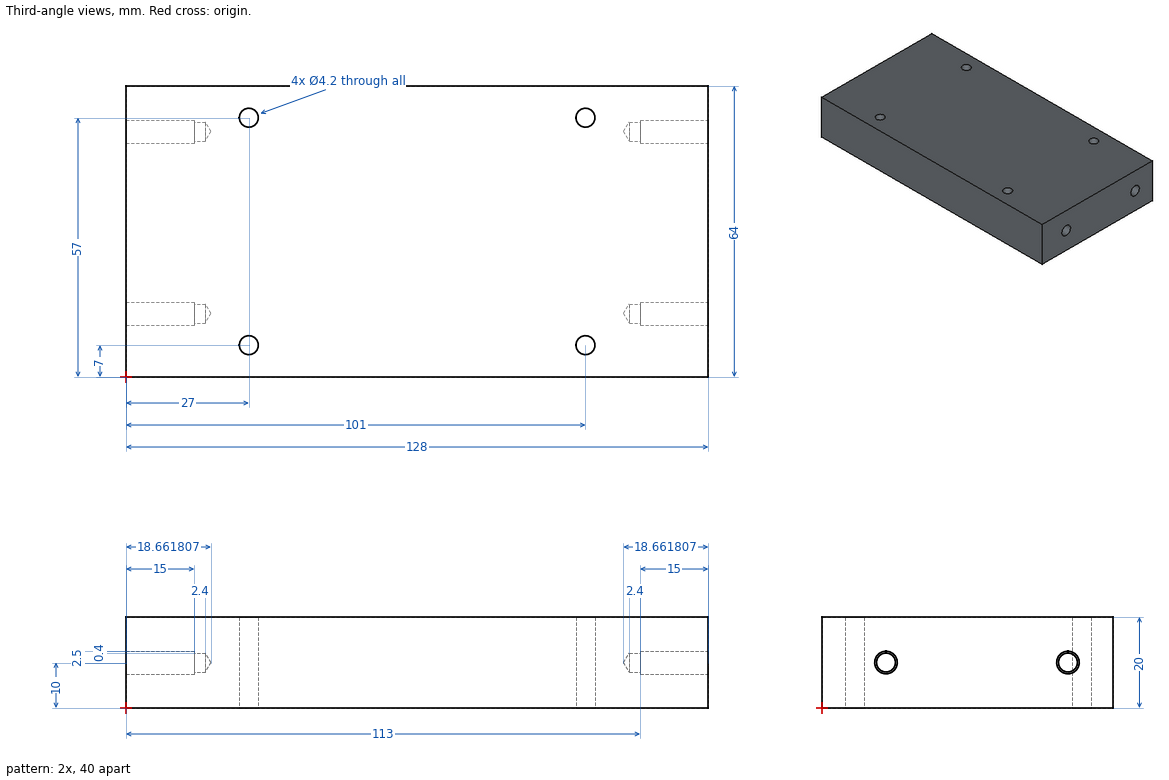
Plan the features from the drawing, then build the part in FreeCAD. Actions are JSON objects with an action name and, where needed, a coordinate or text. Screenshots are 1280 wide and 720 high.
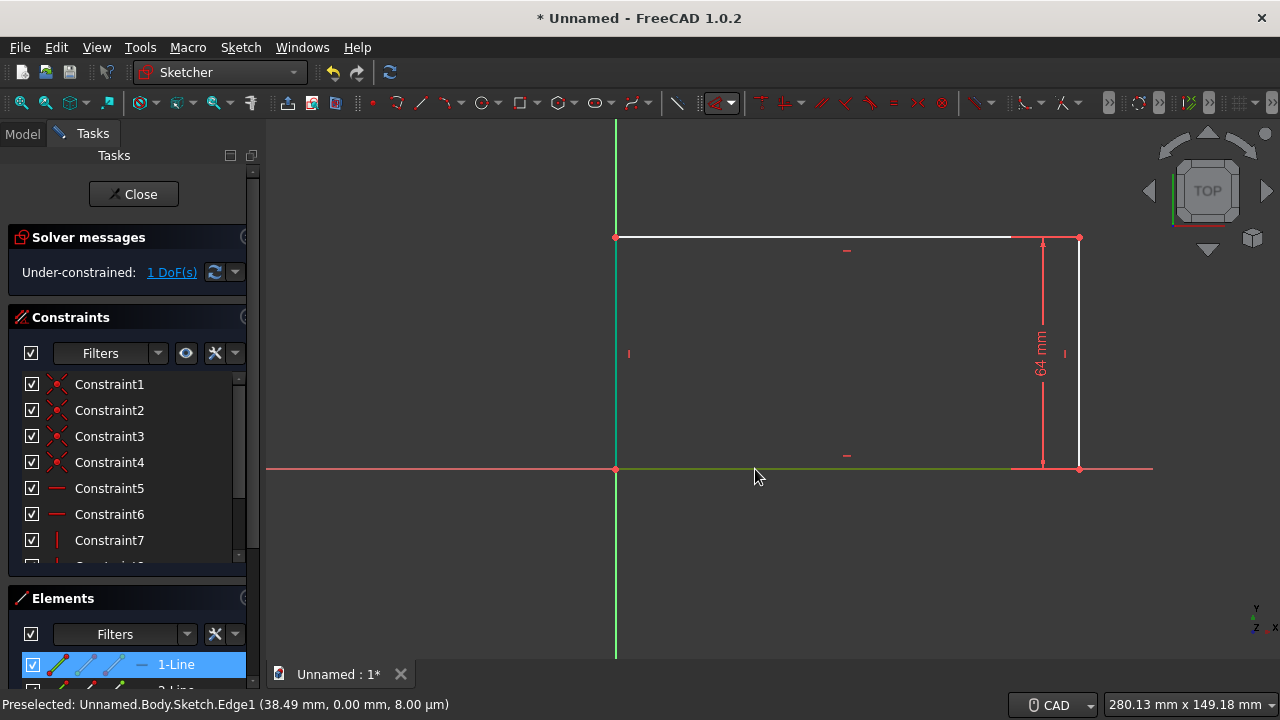
{"action": "left_click", "coordinate": [734, 104]}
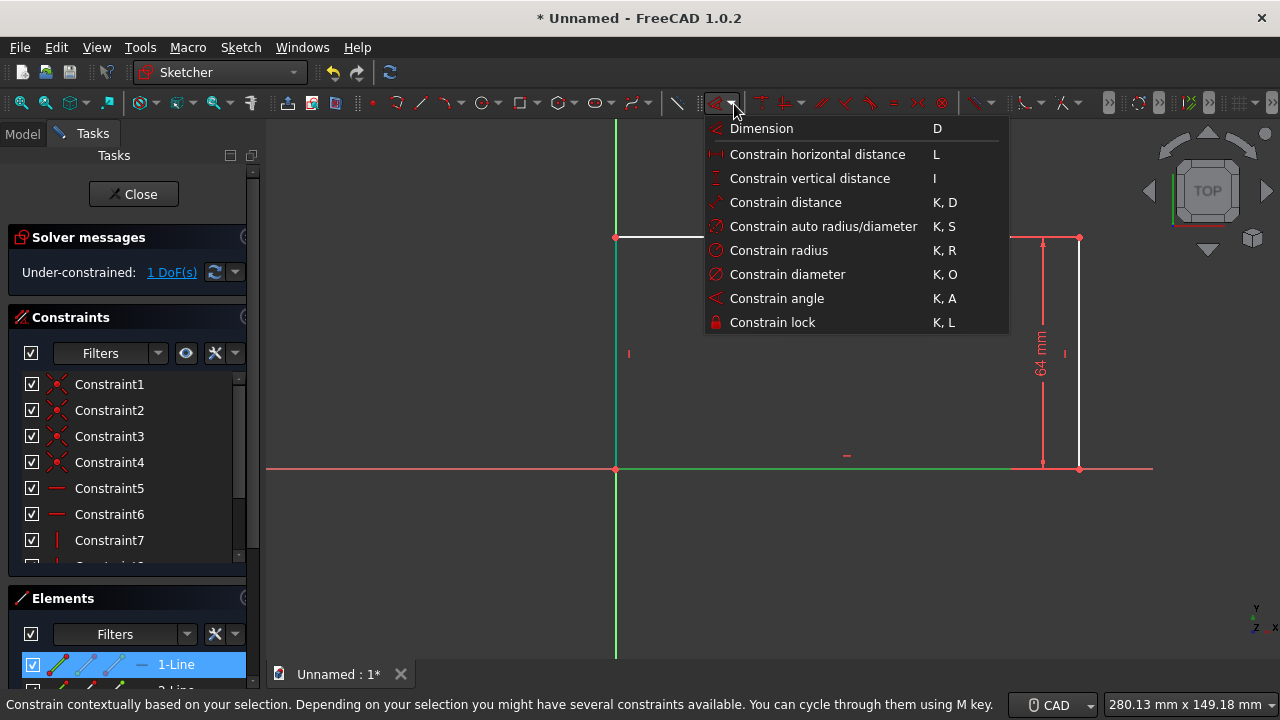
{"action": "left_click", "coordinate": [857, 154]}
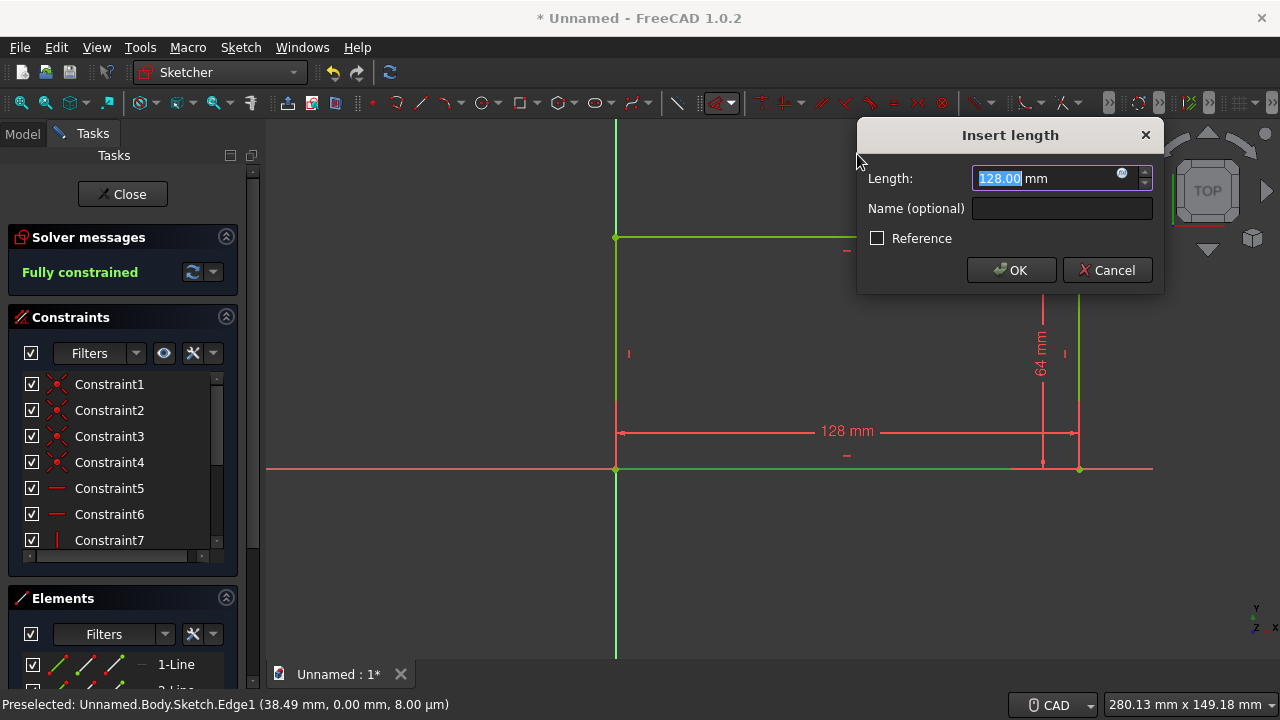
{"action": "type", "text": "128"}
{"action": "key", "text": "Return"}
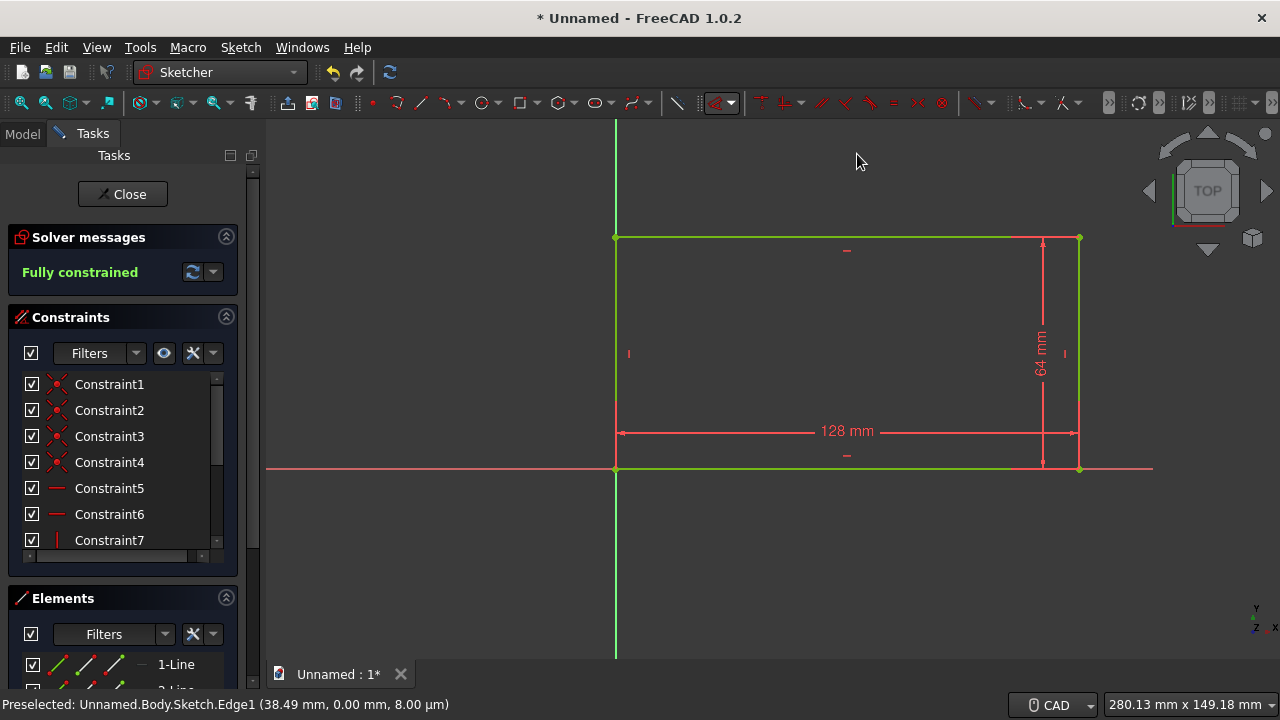
{"action": "left_click", "coordinate": [123, 194]}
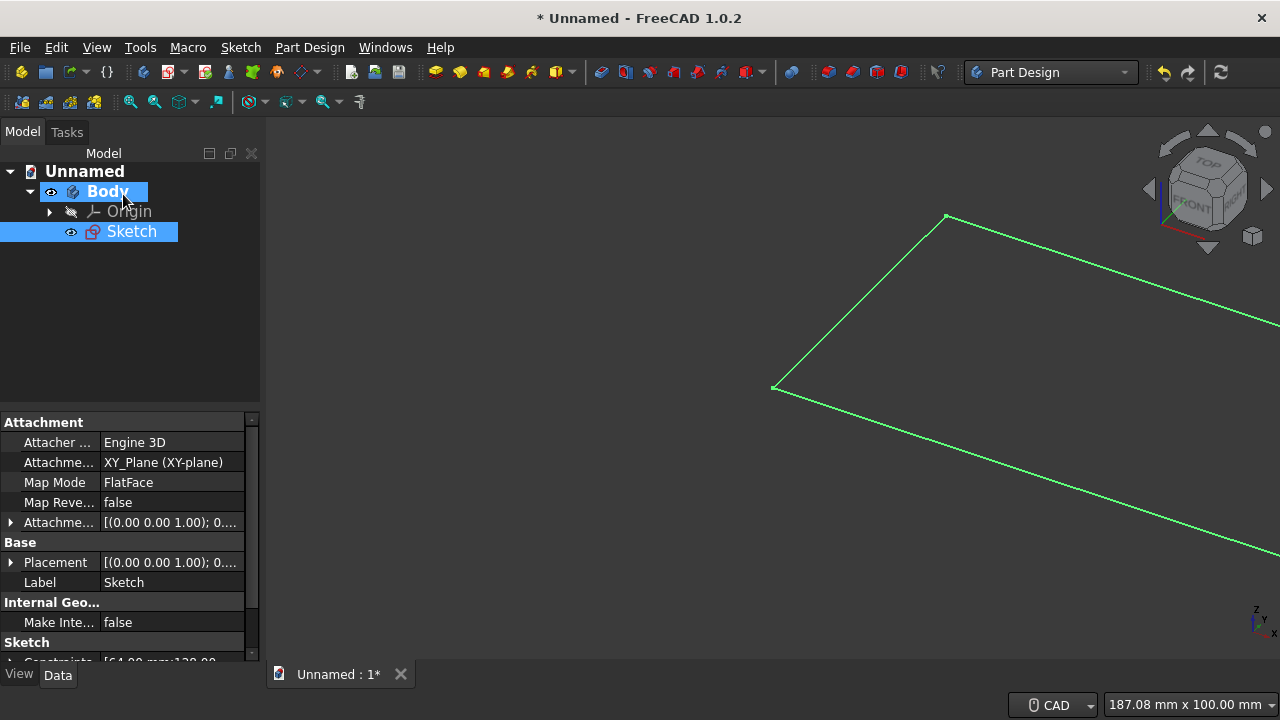
{"action": "left_click", "coordinate": [436, 72]}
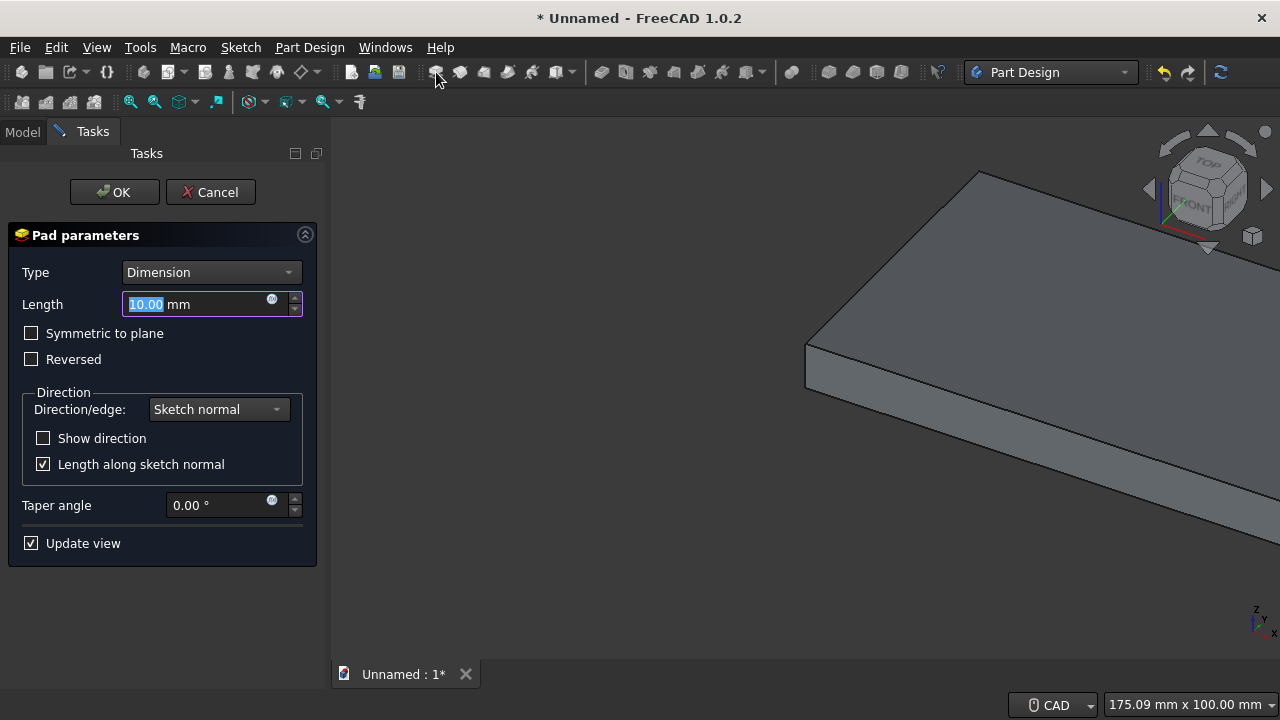
{"action": "type", "text": "20"}
{"action": "key", "text": "Tab"}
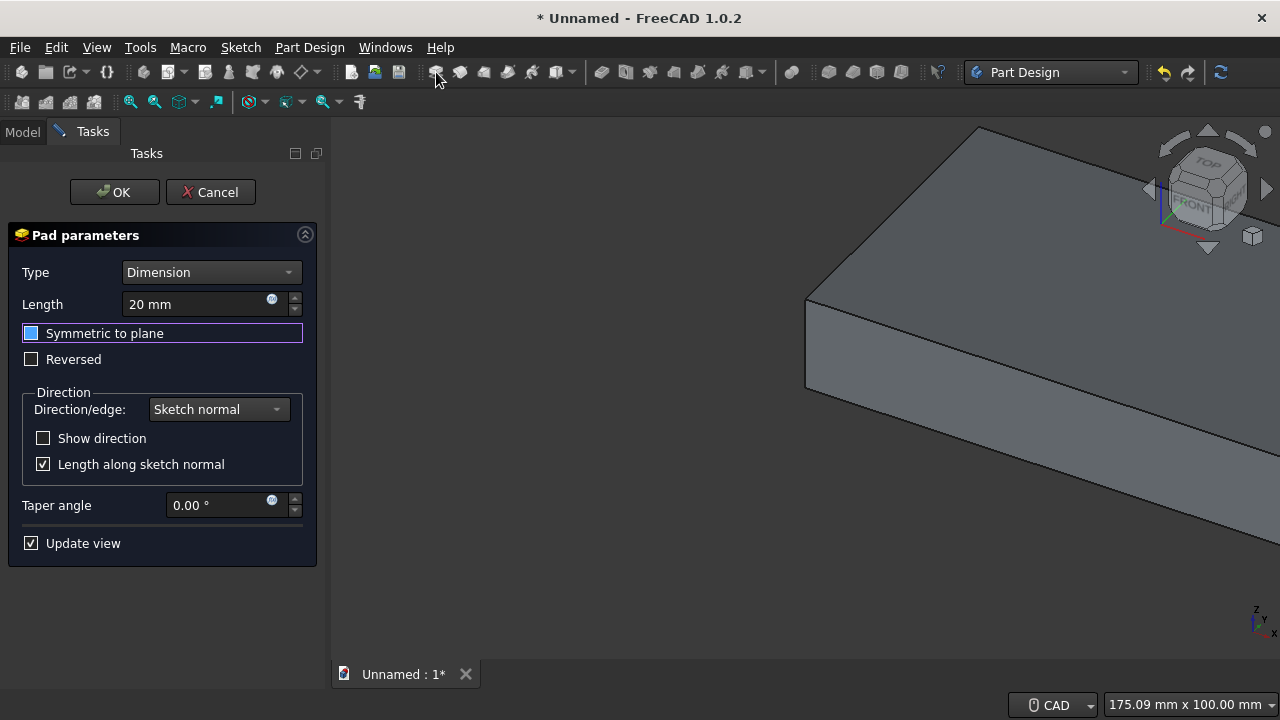
{"action": "left_click", "coordinate": [115, 192]}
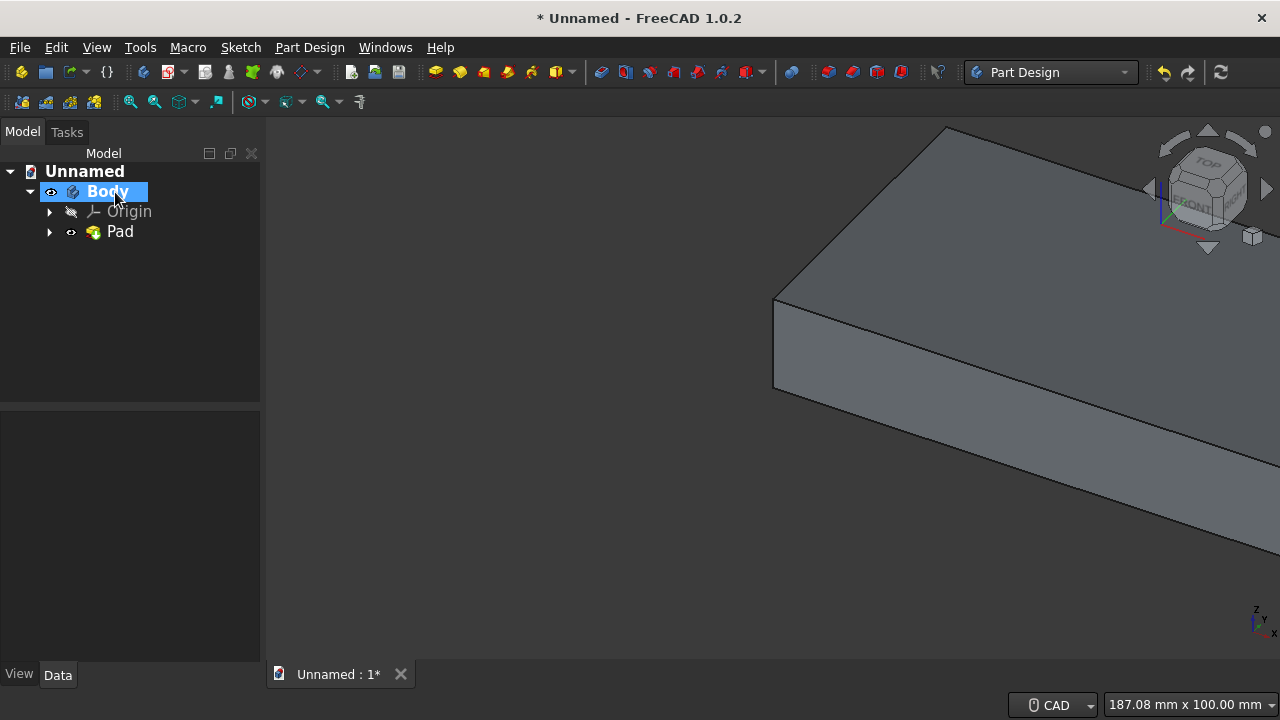
{"action": "left_click", "coordinate": [132, 102]}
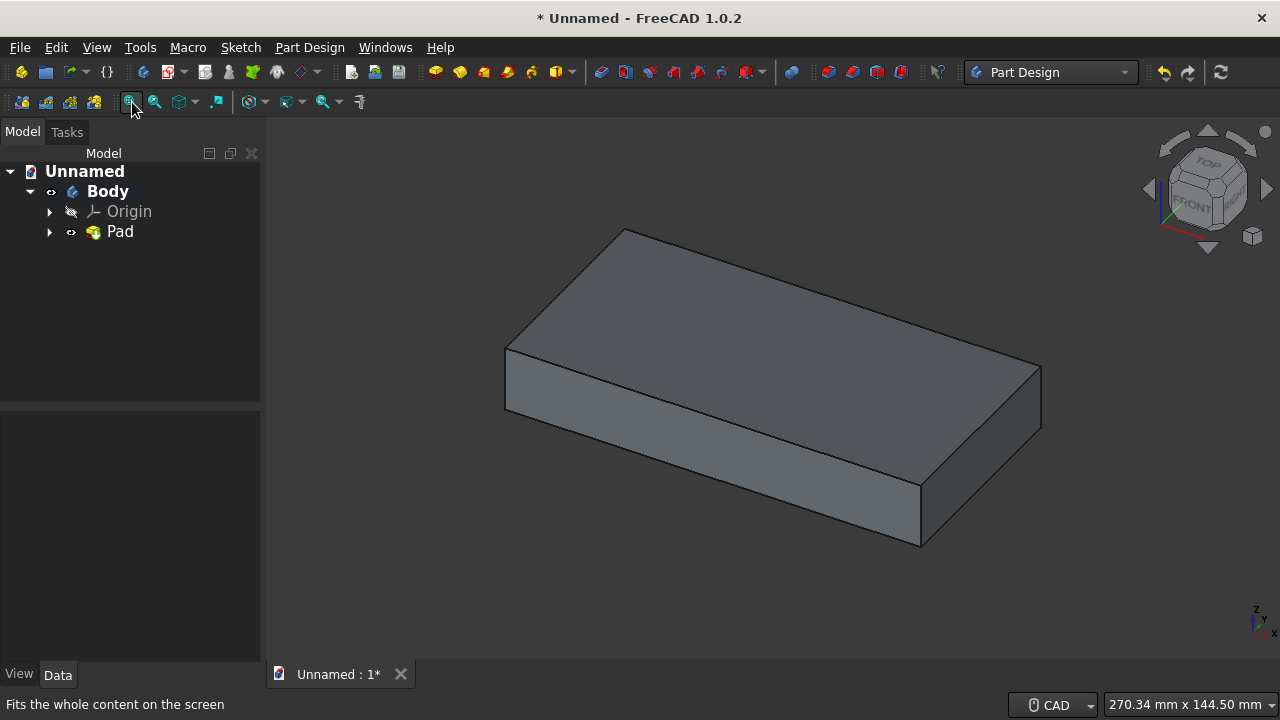
{"action": "left_click", "coordinate": [832, 376]}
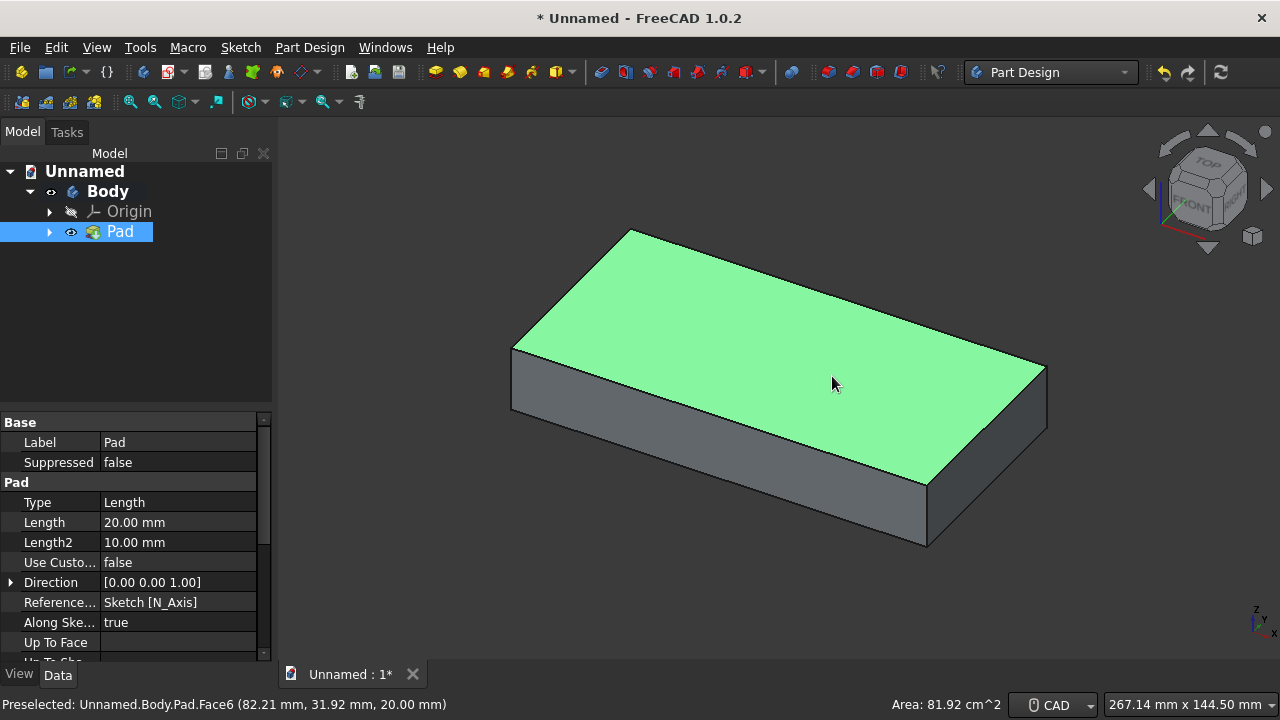
{"action": "left_click", "coordinate": [168, 72]}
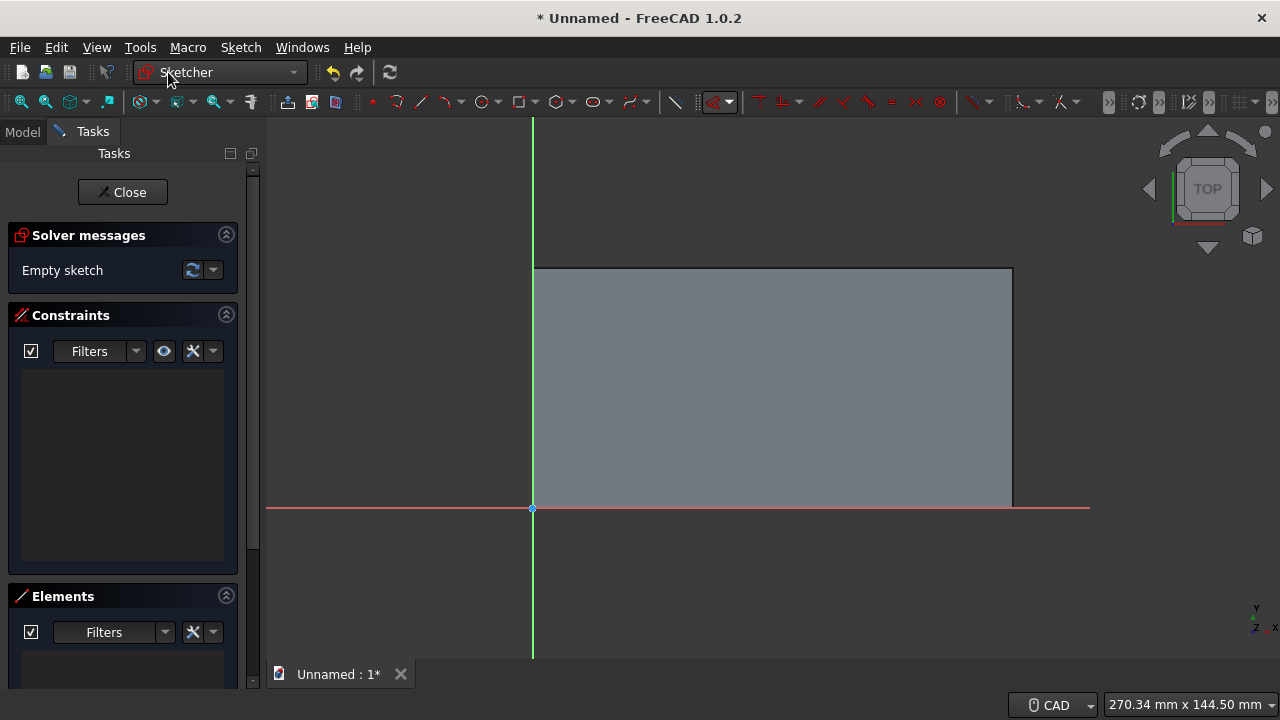
{"action": "scroll", "coordinate": [771, 416], "scroll_direction": "up", "scroll_amount": 2}